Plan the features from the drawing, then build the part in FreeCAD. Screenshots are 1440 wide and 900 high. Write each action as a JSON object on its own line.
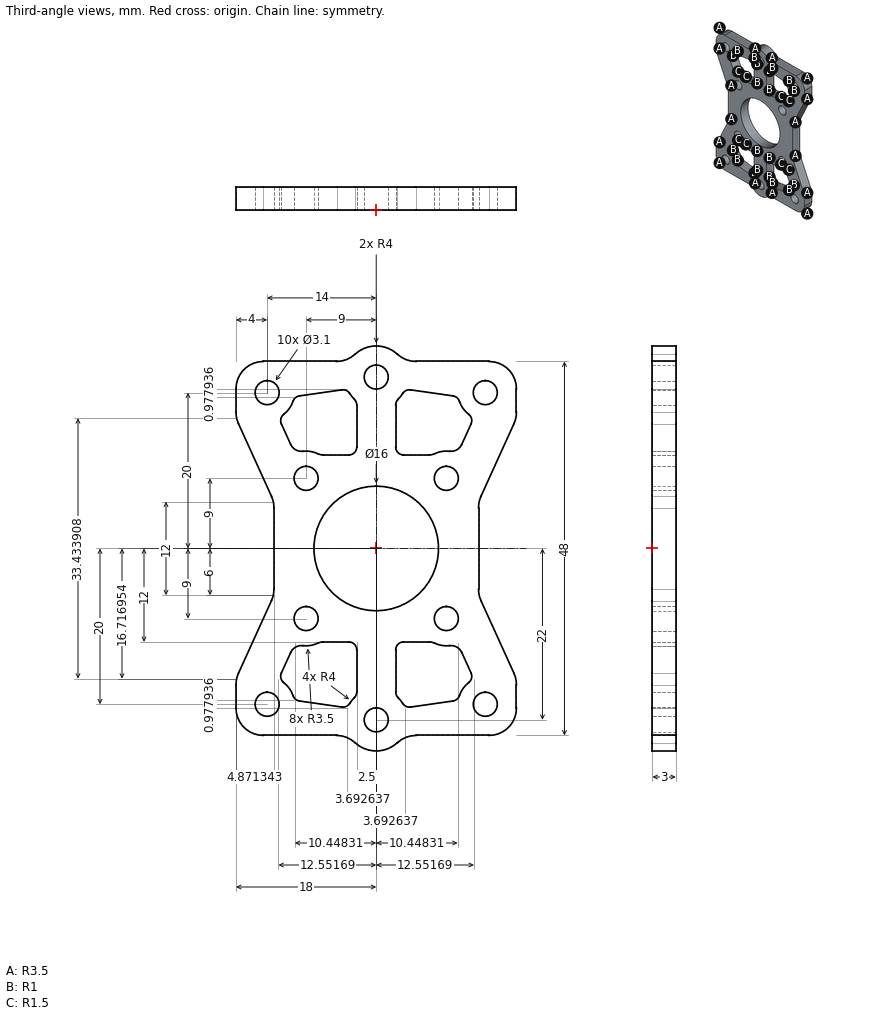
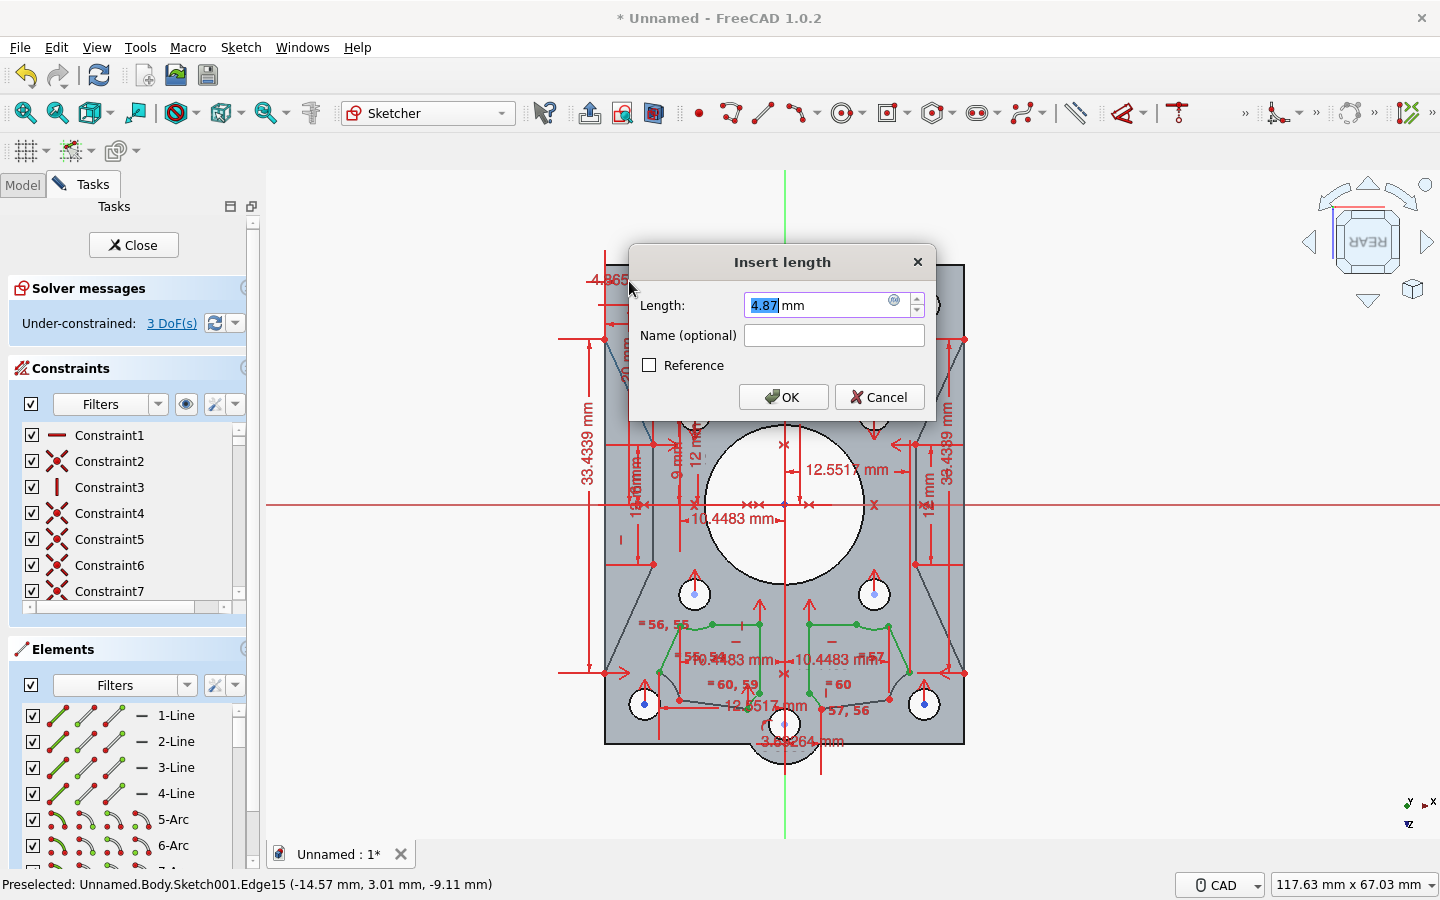
{"action": "type", "text": "4.871343"}
{"action": "key", "text": "Return"}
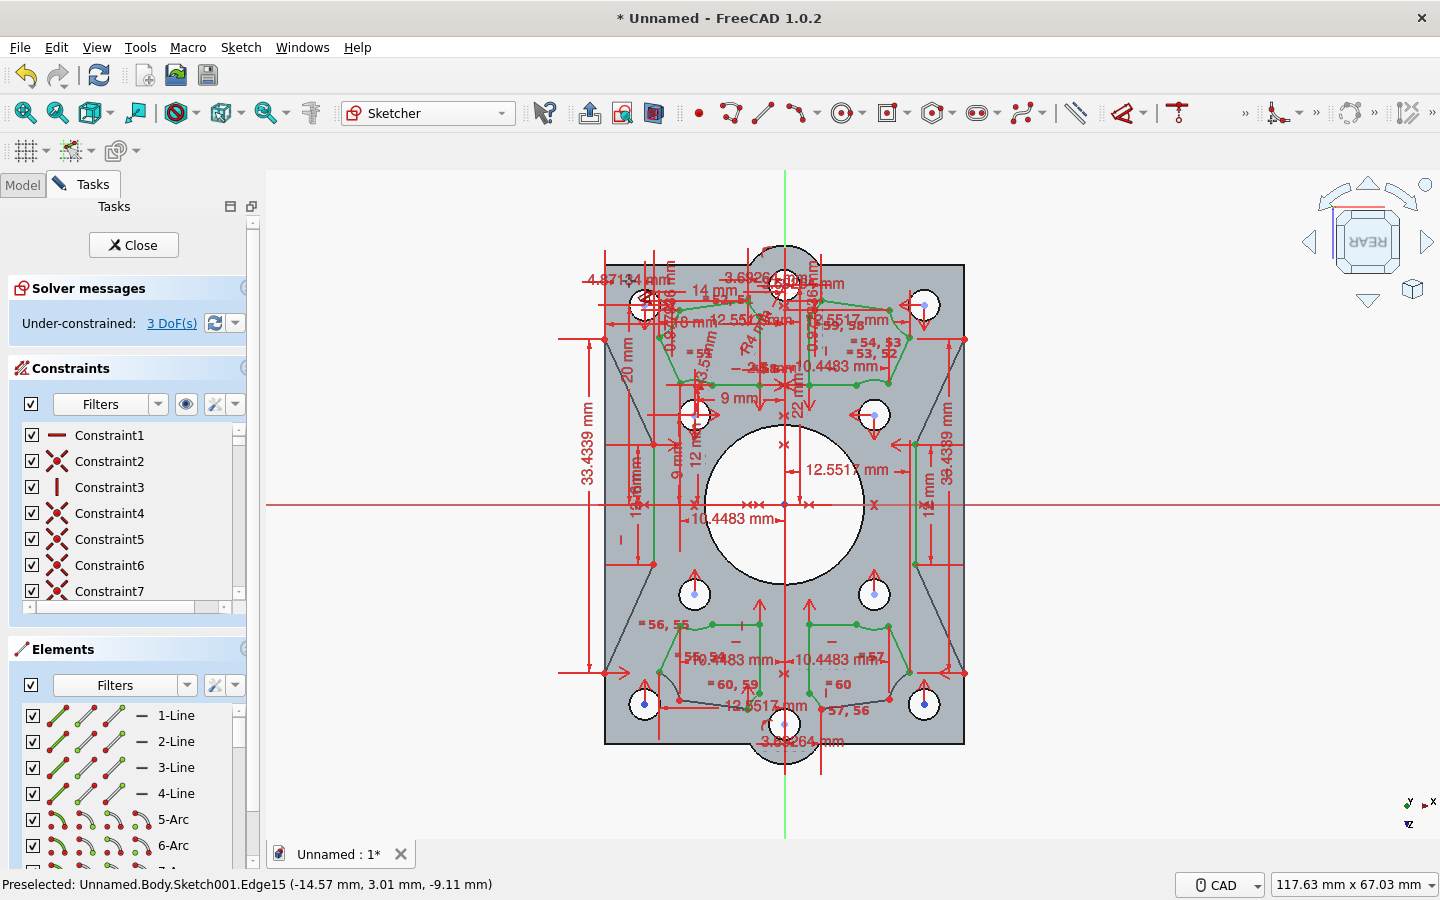
{"action": "scroll", "coordinate": [700, 703], "scroll_direction": "up", "scroll_amount": 8}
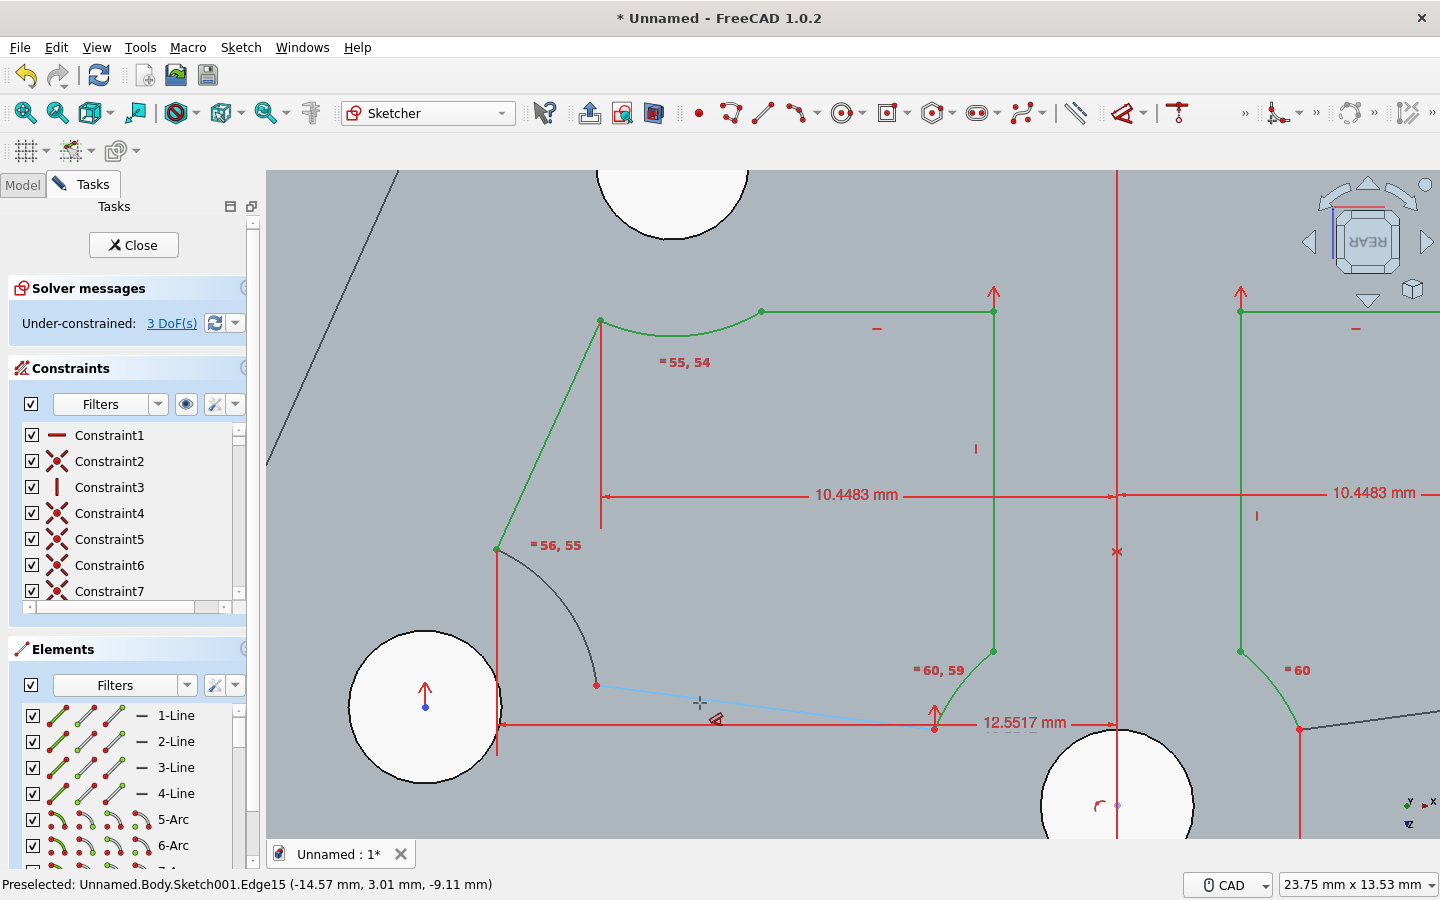
{"action": "left_click", "coordinate": [698, 699]}
{"action": "left_click", "coordinate": [563, 708]}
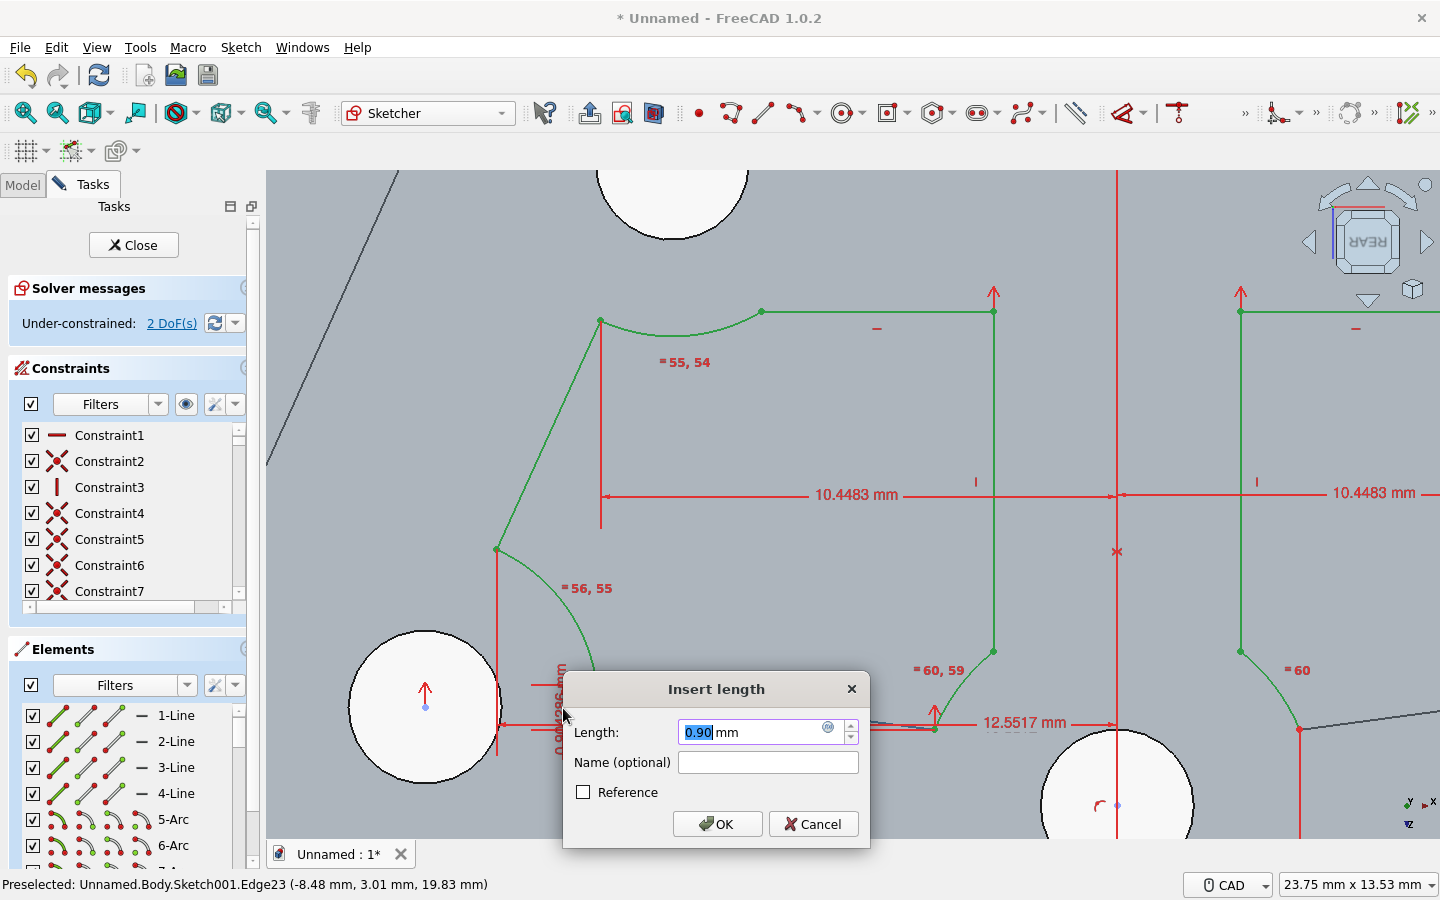
{"action": "type", "text": "0.977936"}
{"action": "key", "text": "Return"}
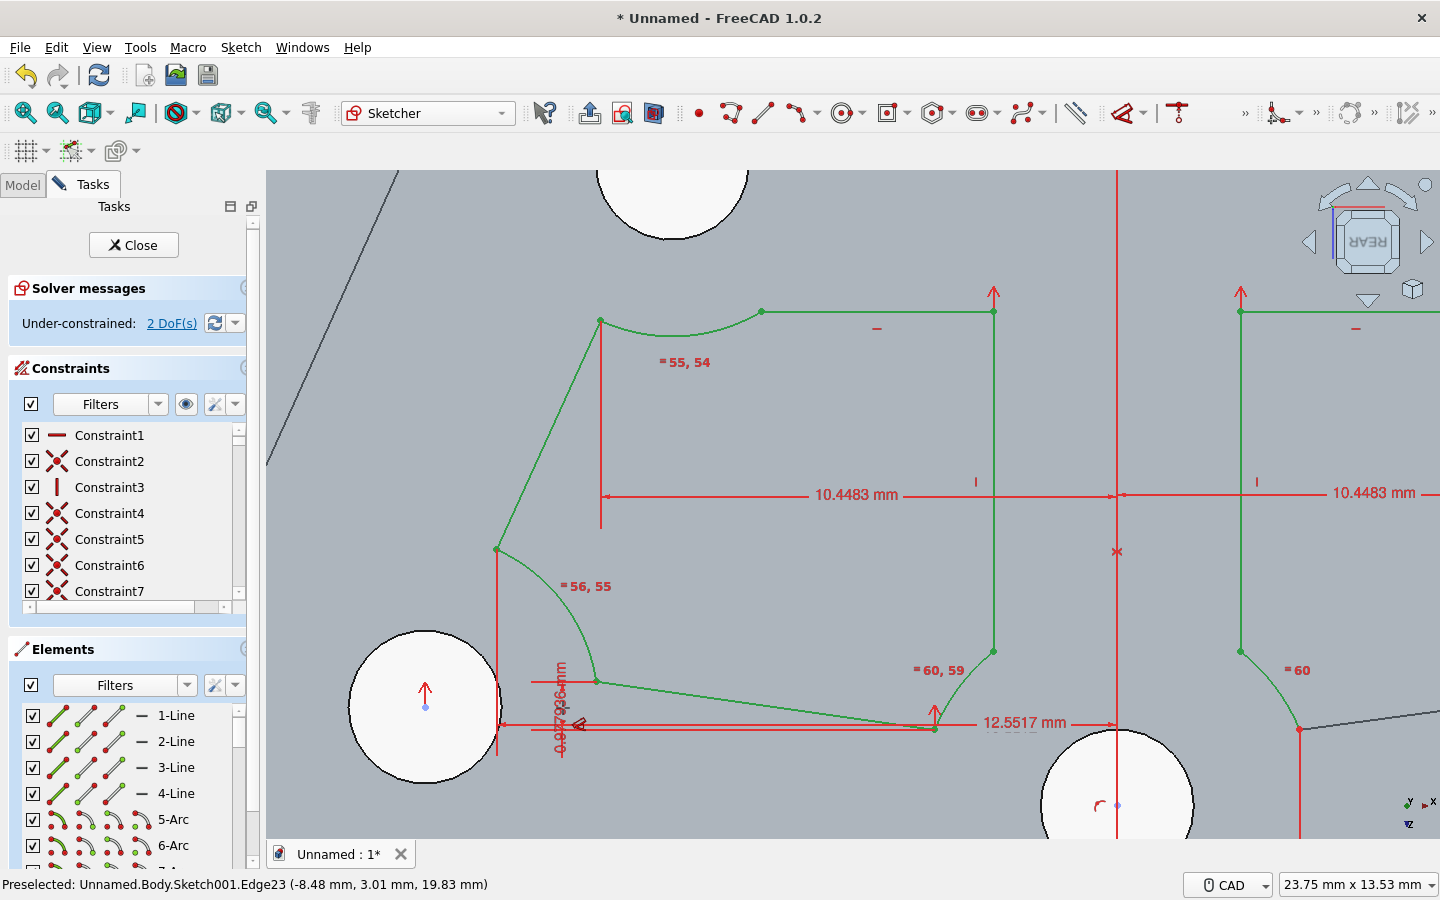
{"action": "scroll", "coordinate": [700, 703], "scroll_direction": "down", "scroll_amount": 8}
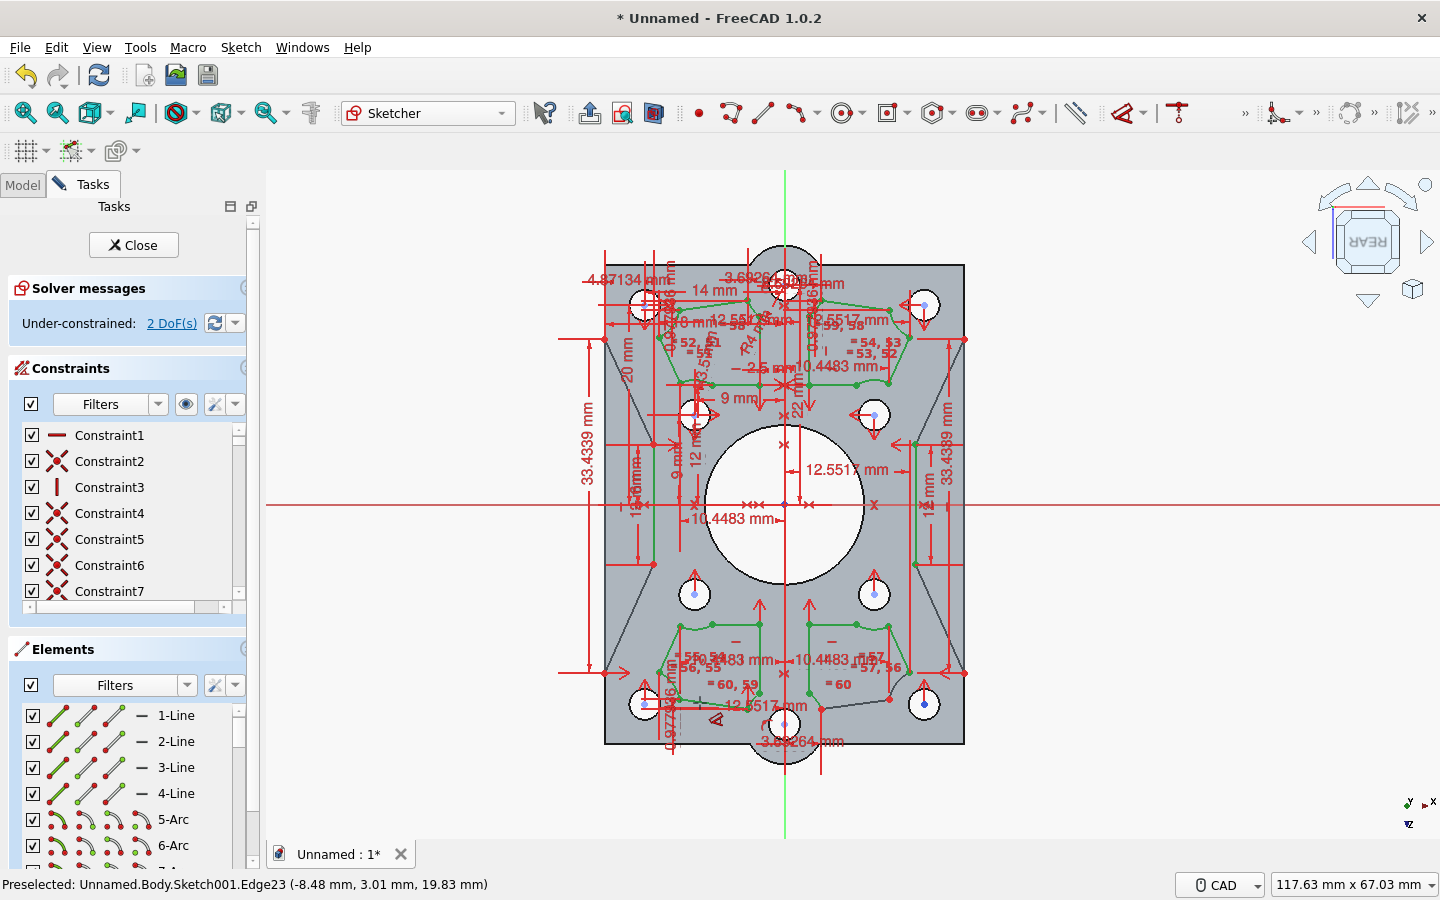
{"action": "scroll", "coordinate": [842, 706], "scroll_direction": "up", "scroll_amount": 8}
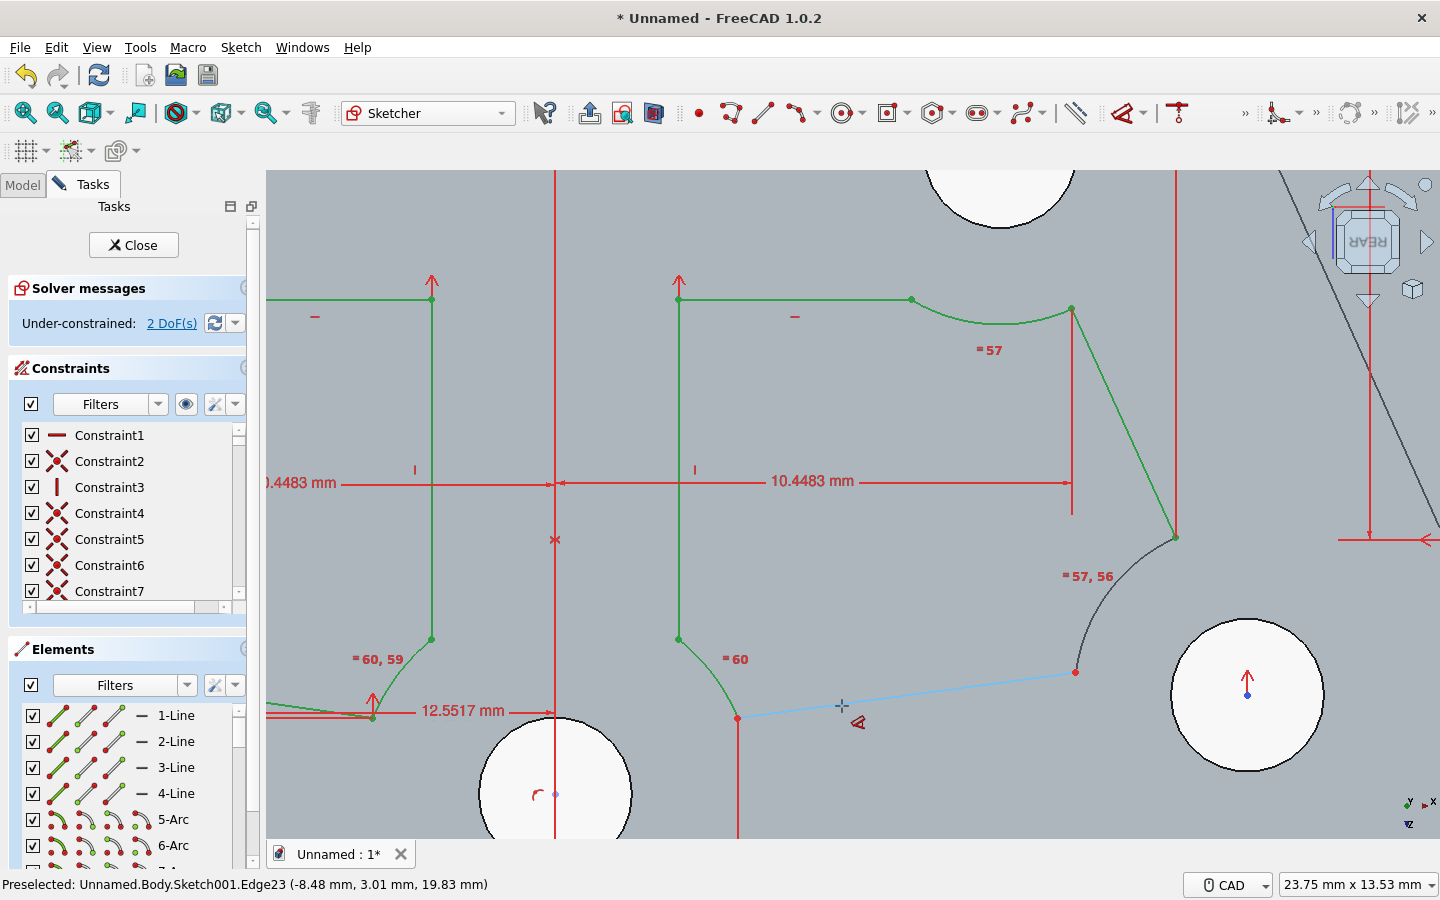
{"action": "left_click", "coordinate": [839, 704]}
{"action": "left_click", "coordinate": [1110, 695]}